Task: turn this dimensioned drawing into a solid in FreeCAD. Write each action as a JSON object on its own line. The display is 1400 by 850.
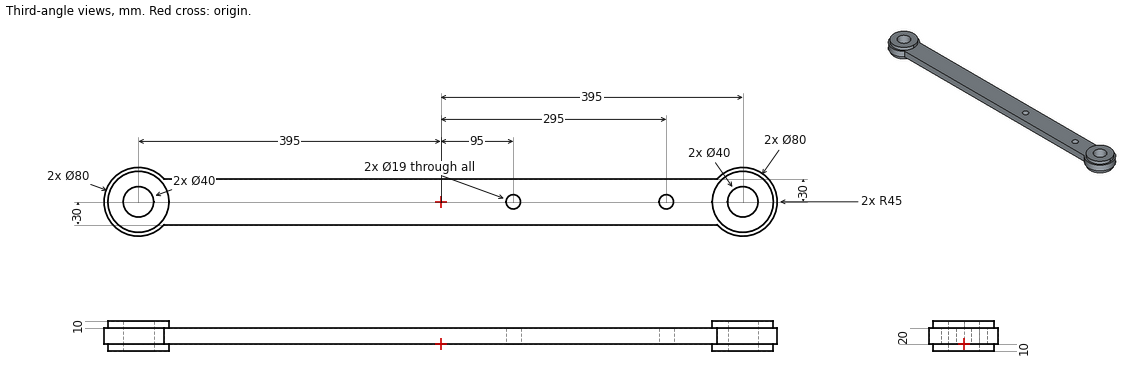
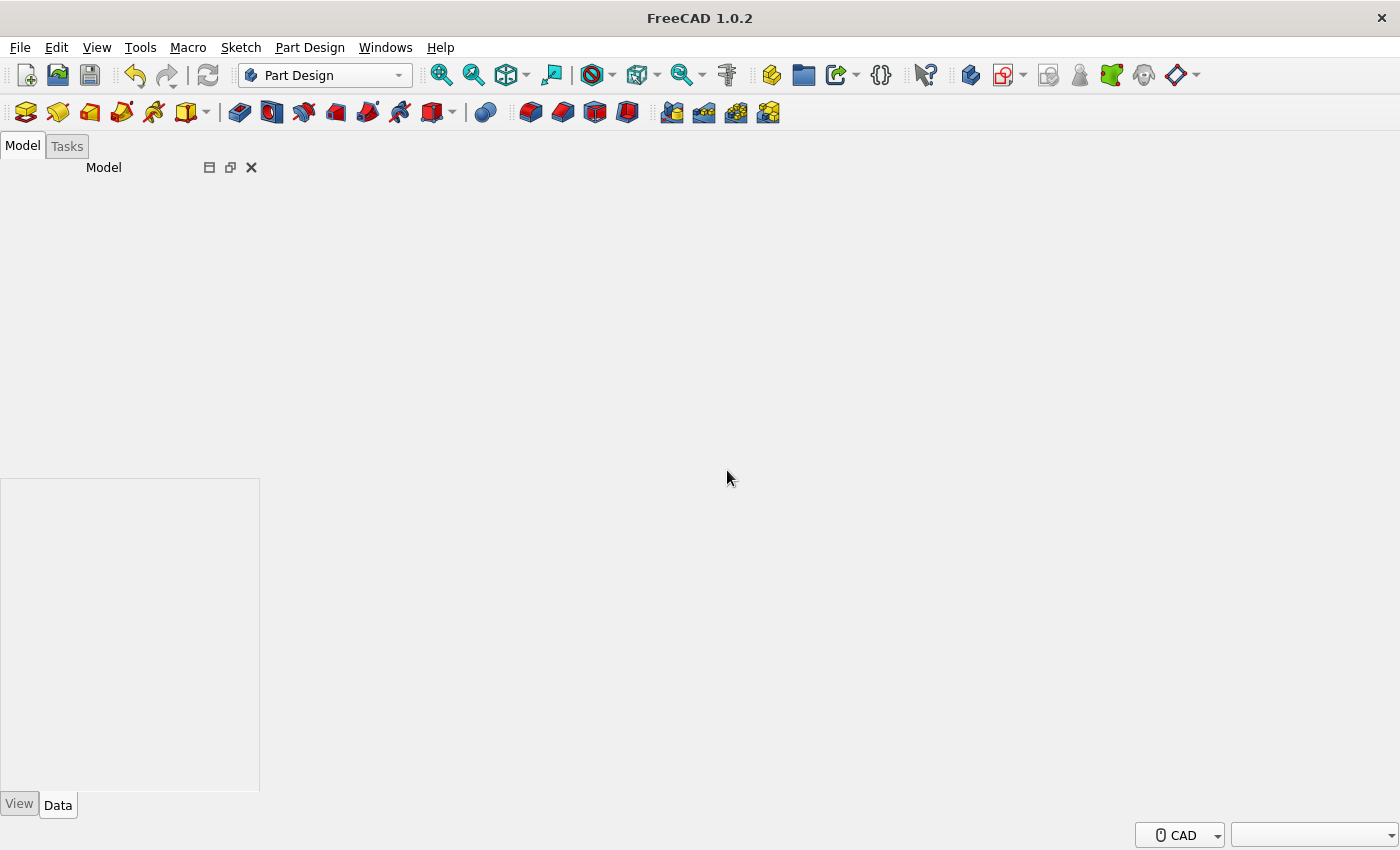
{"action": "left_click", "coordinate": [26, 76]}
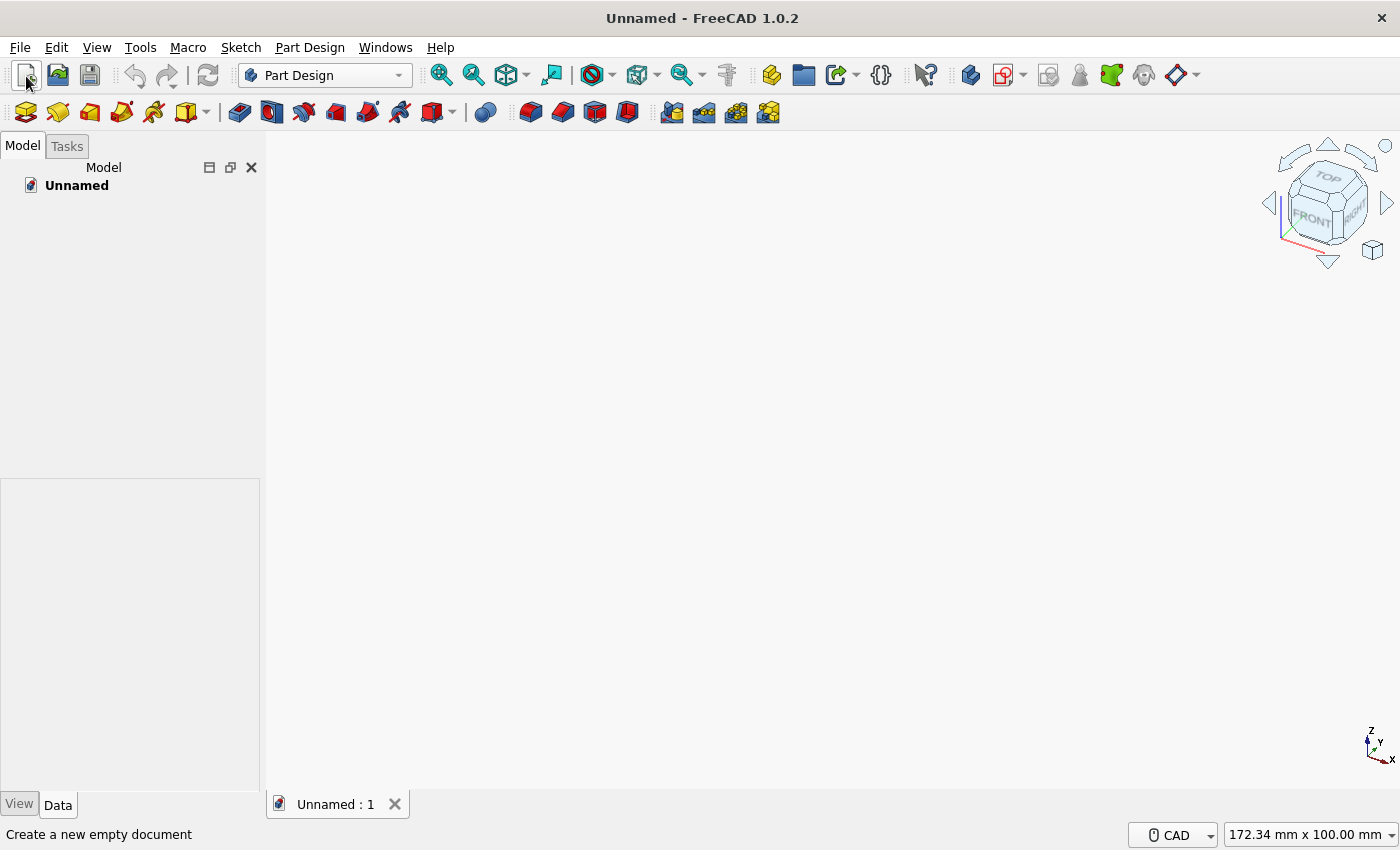
{"action": "left_click", "coordinate": [1004, 76]}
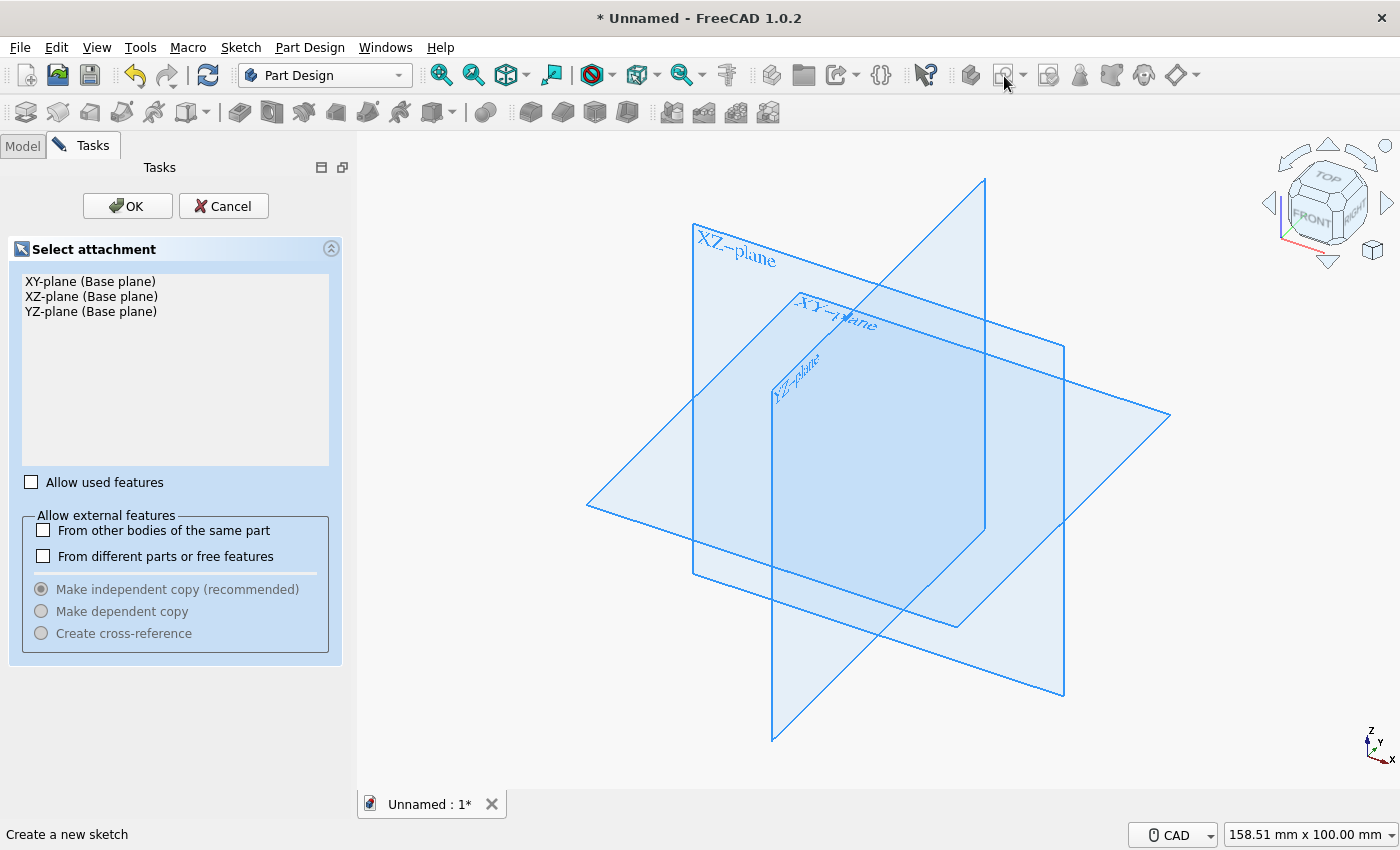
{"action": "left_click", "coordinate": [82, 282]}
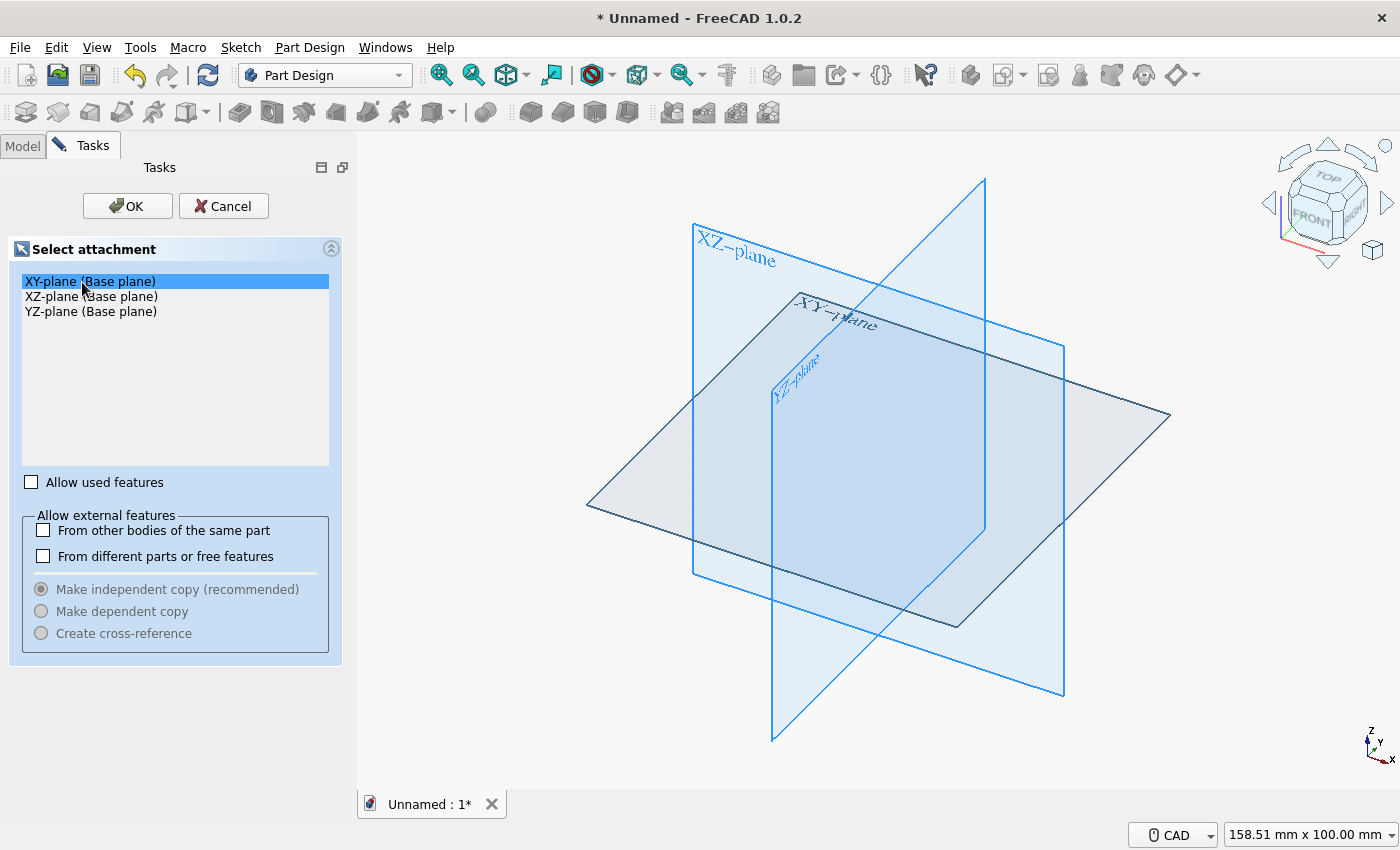
{"action": "left_click", "coordinate": [128, 206]}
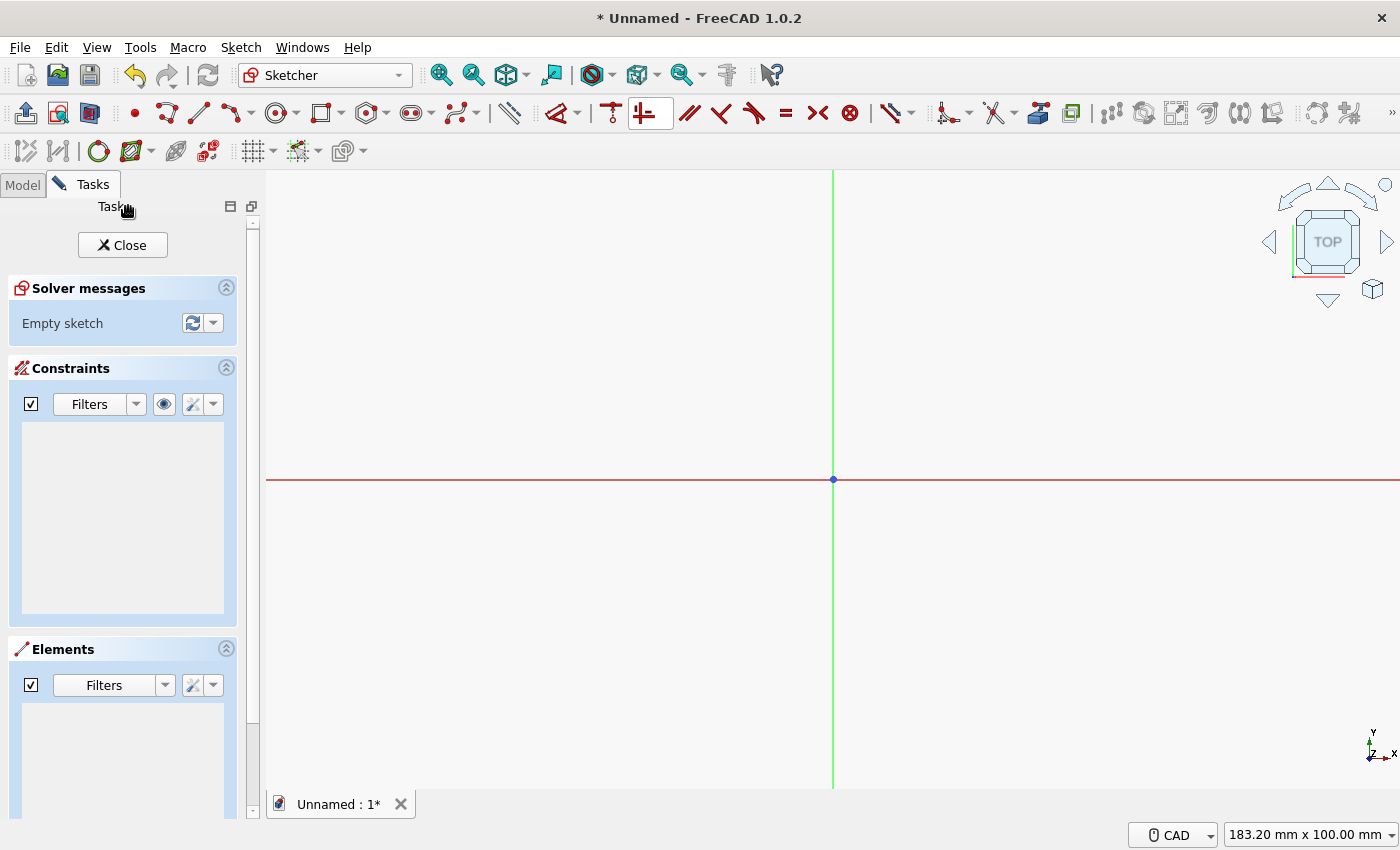
{"action": "scroll", "coordinate": [756, 480], "scroll_direction": "down", "scroll_amount": 11}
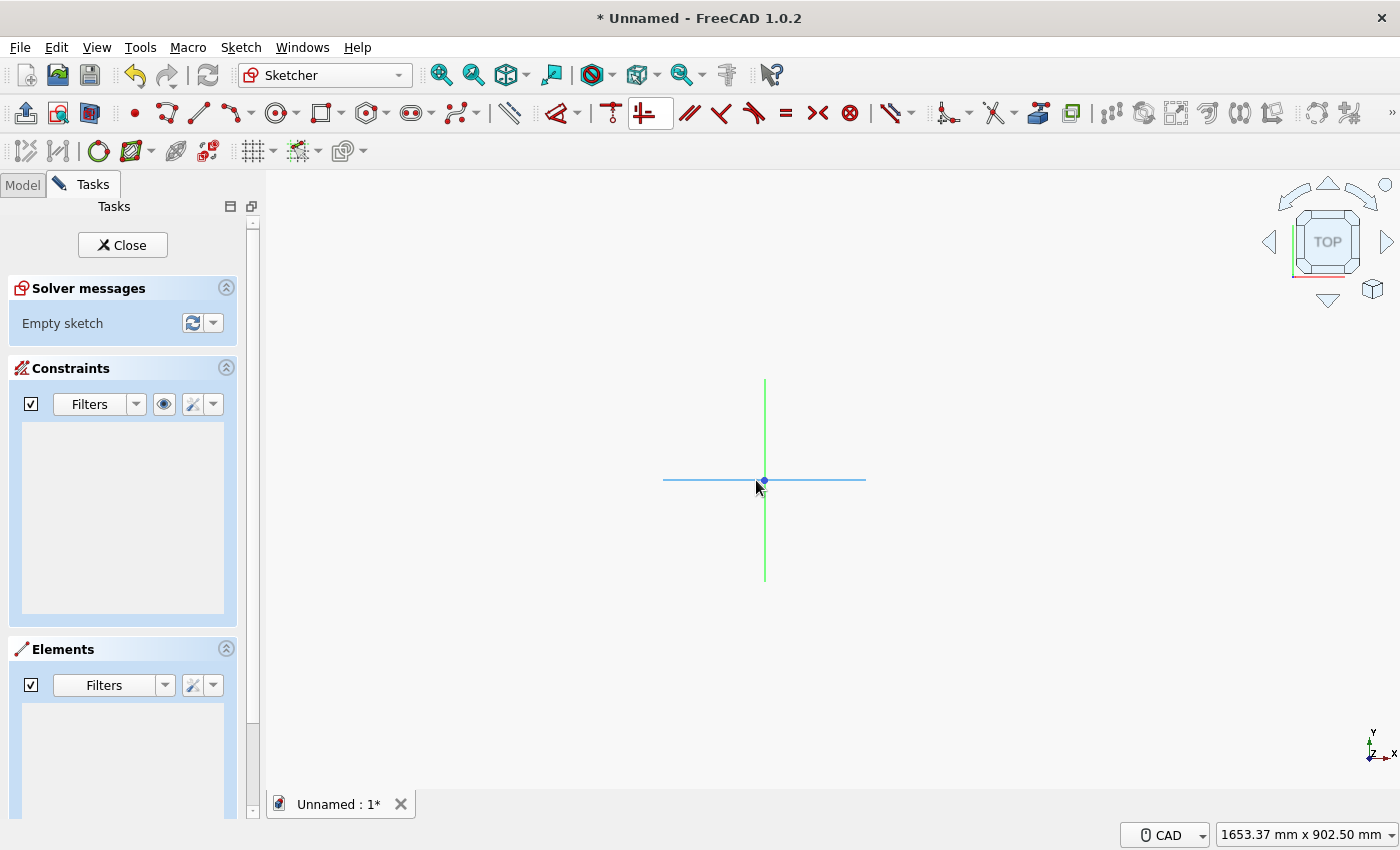
{"action": "left_click", "coordinate": [200, 114]}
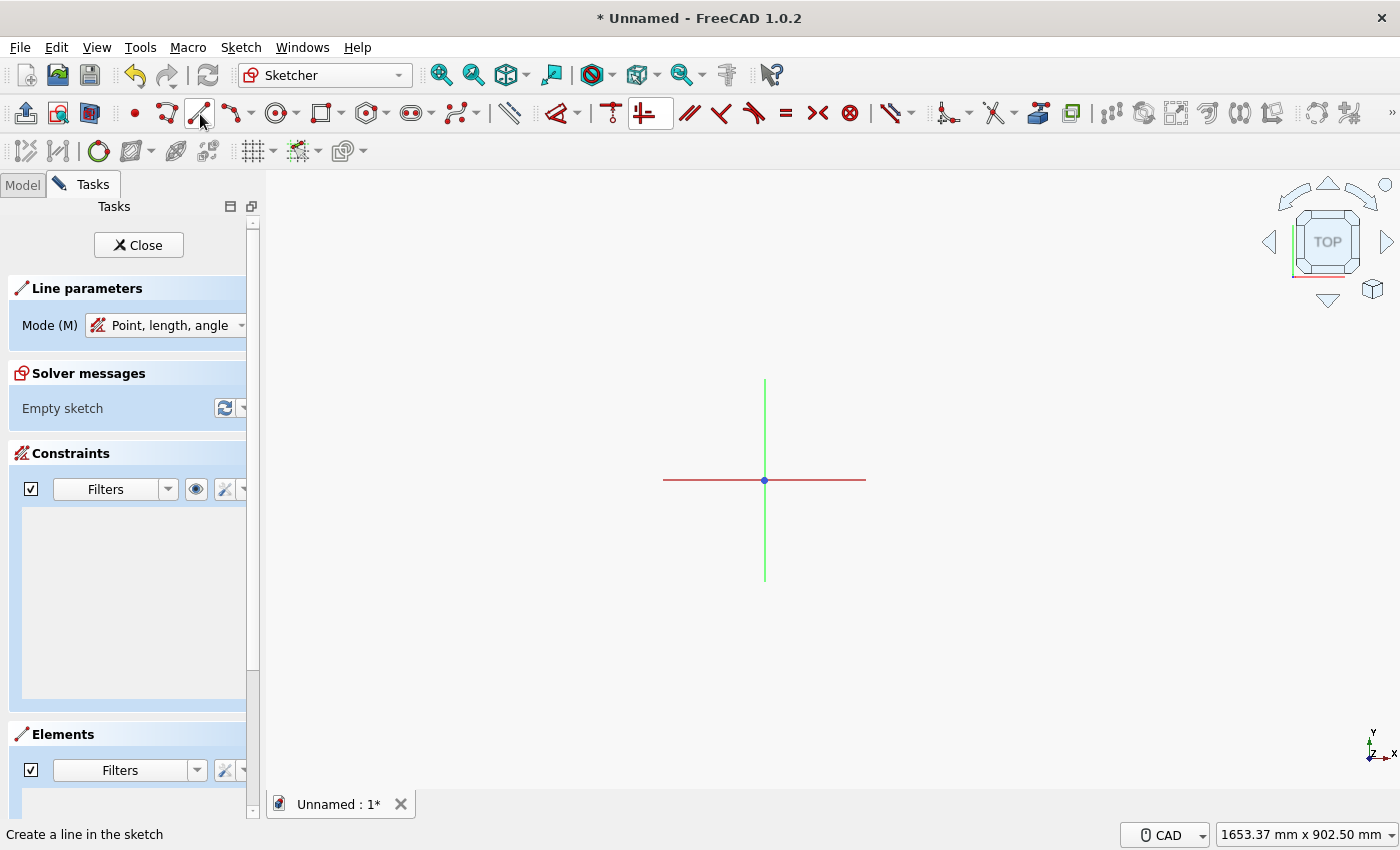
{"action": "left_click", "coordinate": [1013, 460]}
{"action": "left_click", "coordinate": [517, 460]}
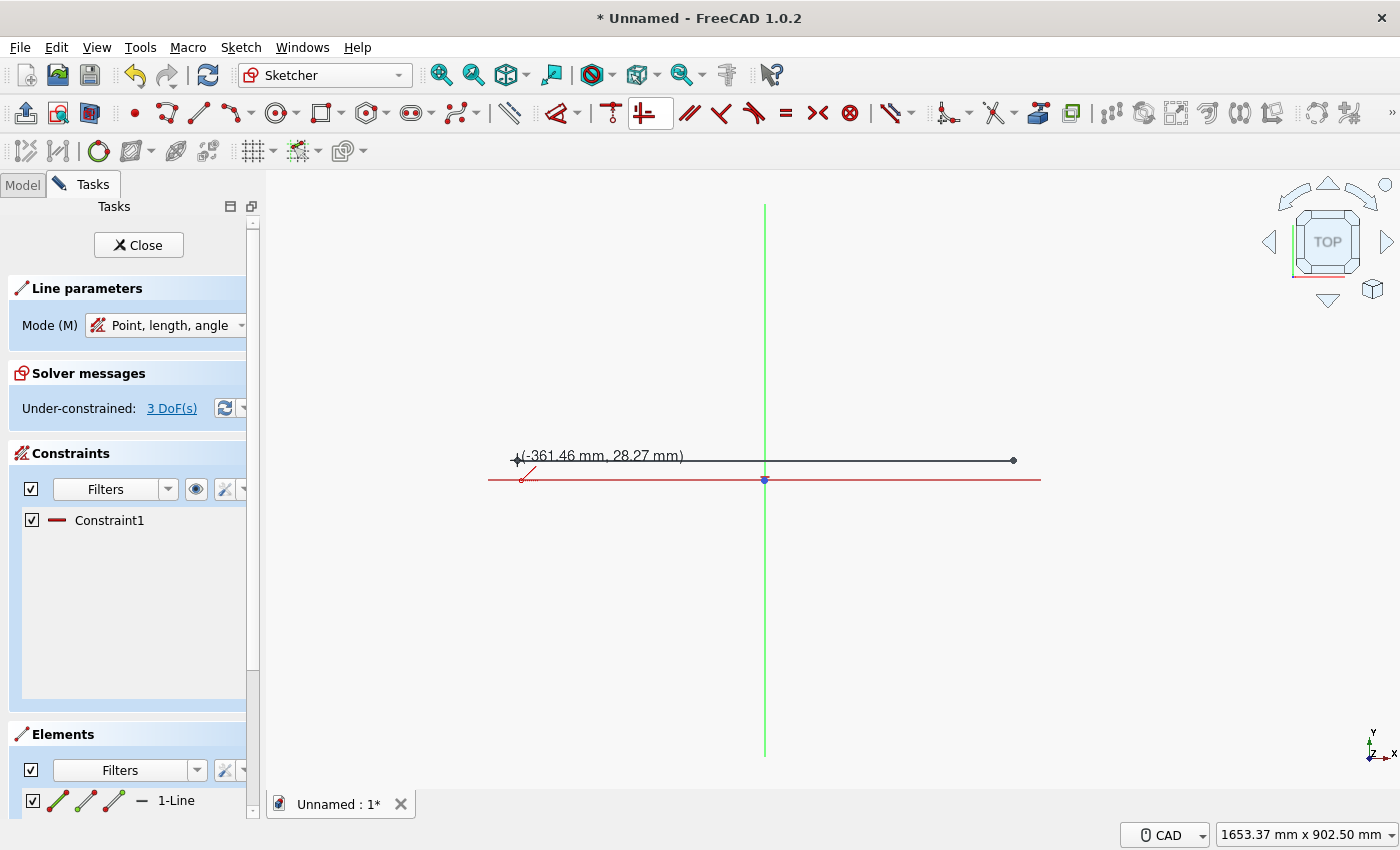
{"action": "left_click", "coordinate": [517, 501]}
{"action": "left_click", "coordinate": [1013, 501]}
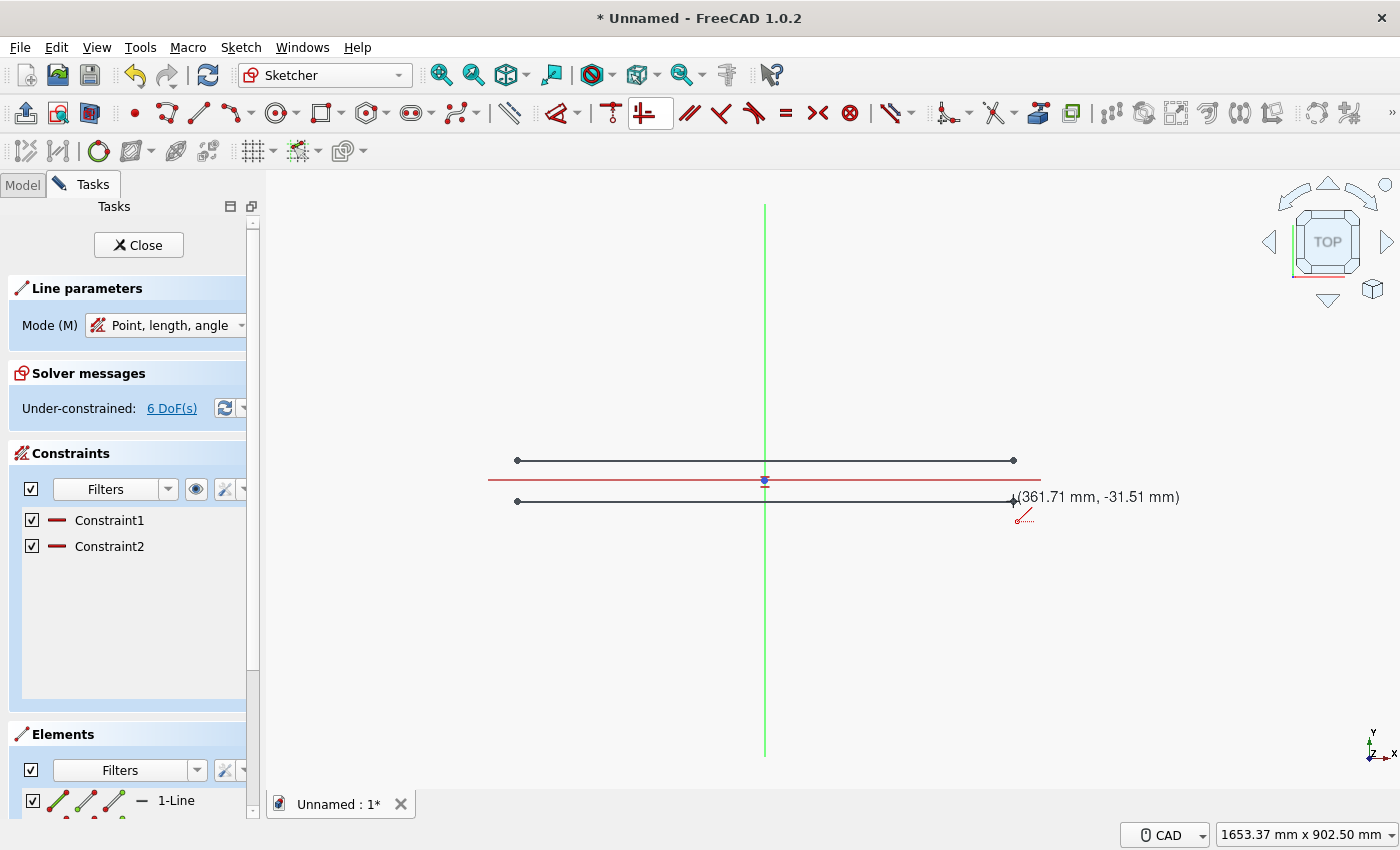
{"action": "left_click", "coordinate": [232, 114]}